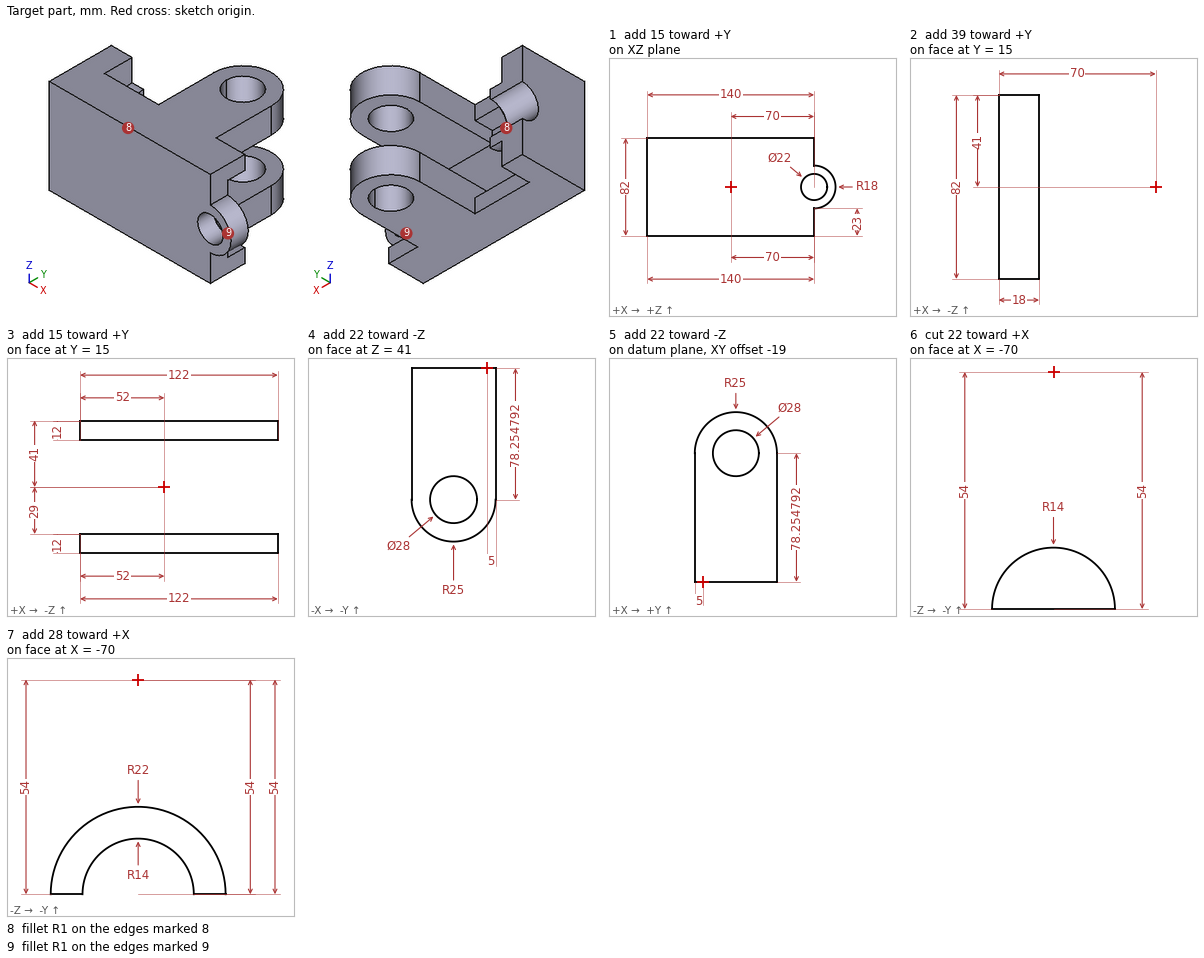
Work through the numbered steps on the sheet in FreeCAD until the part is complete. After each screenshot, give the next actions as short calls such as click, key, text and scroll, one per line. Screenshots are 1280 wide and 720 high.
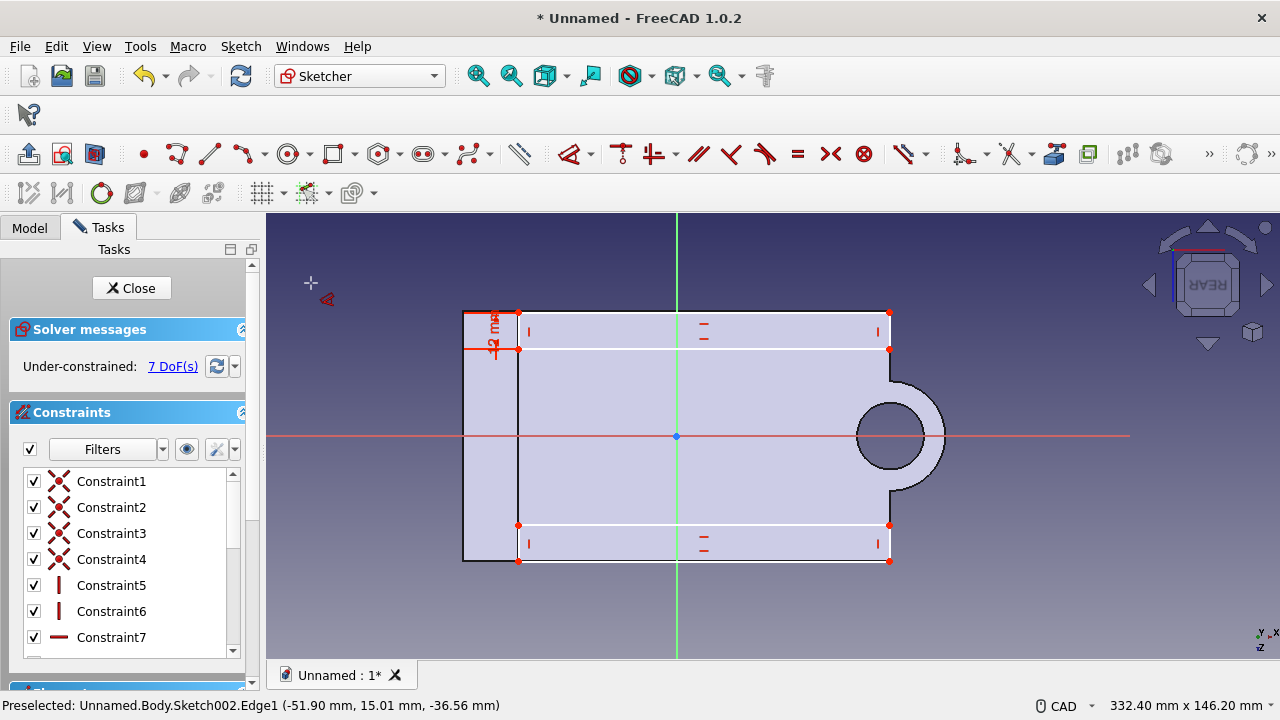
scroll(519, 536, up, 2)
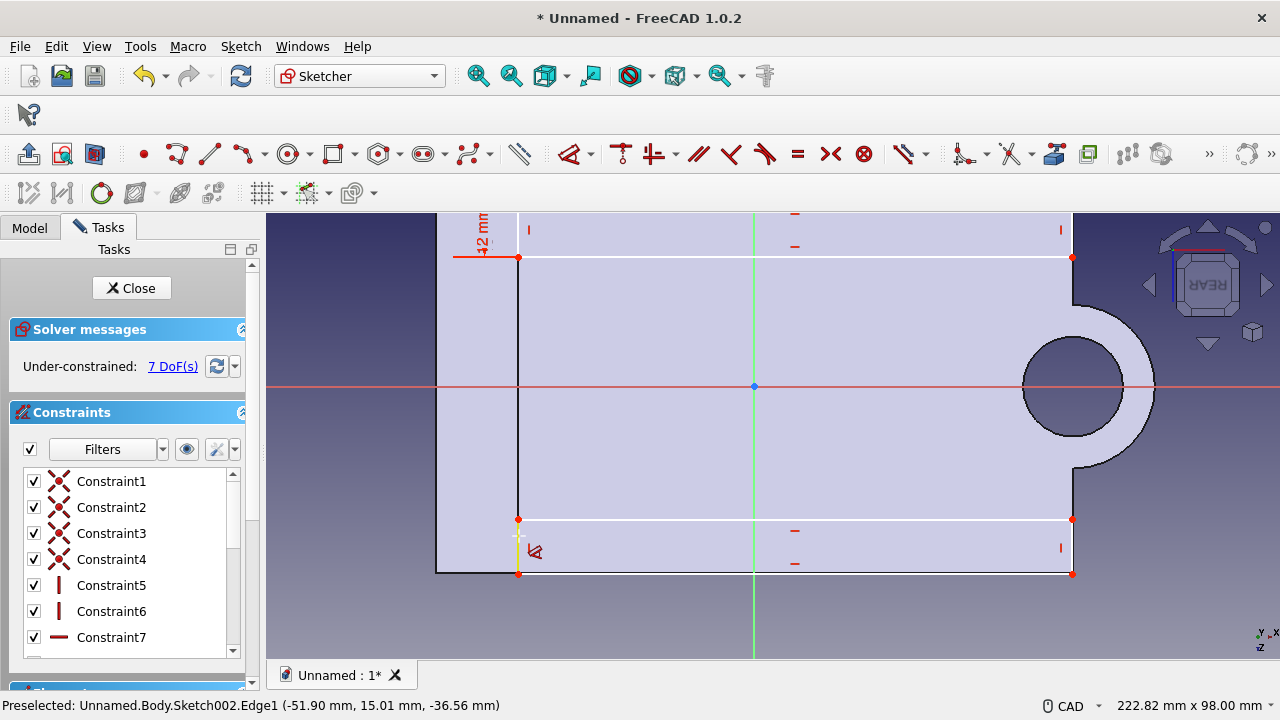
click(518, 536)
click(484, 547)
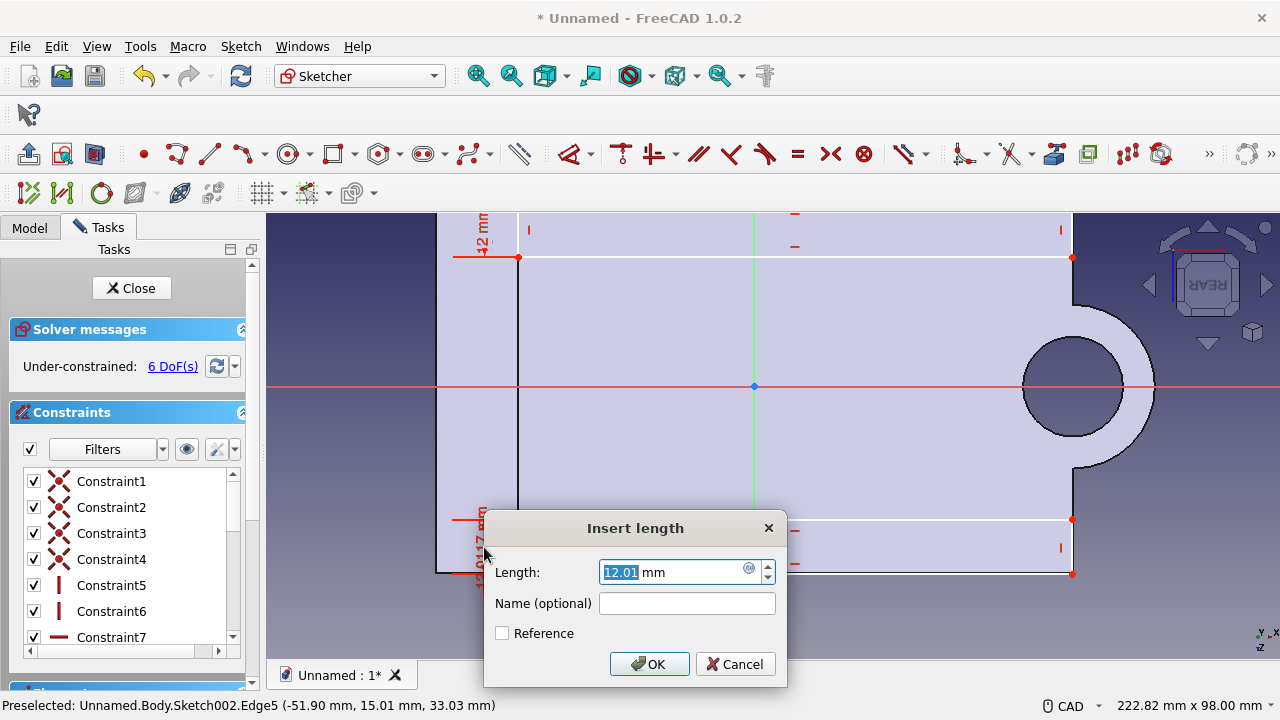
text(12)
key(Return)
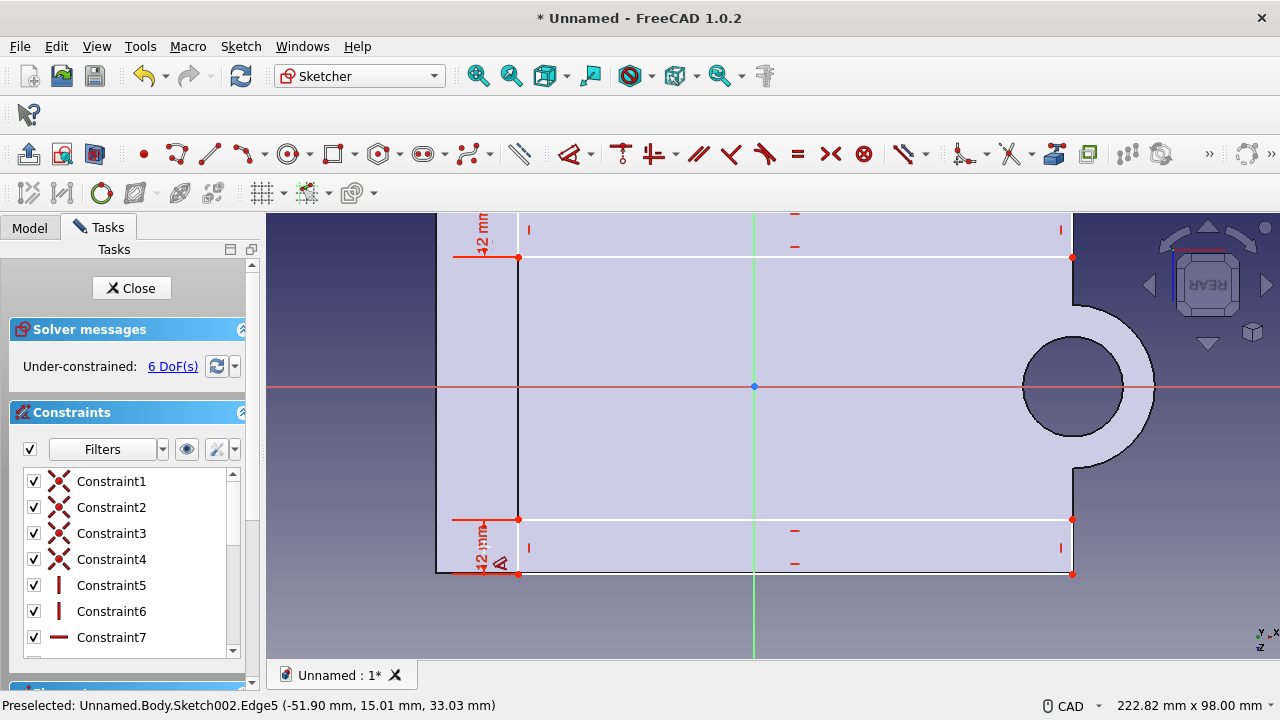
click(684, 257)
click(795, 291)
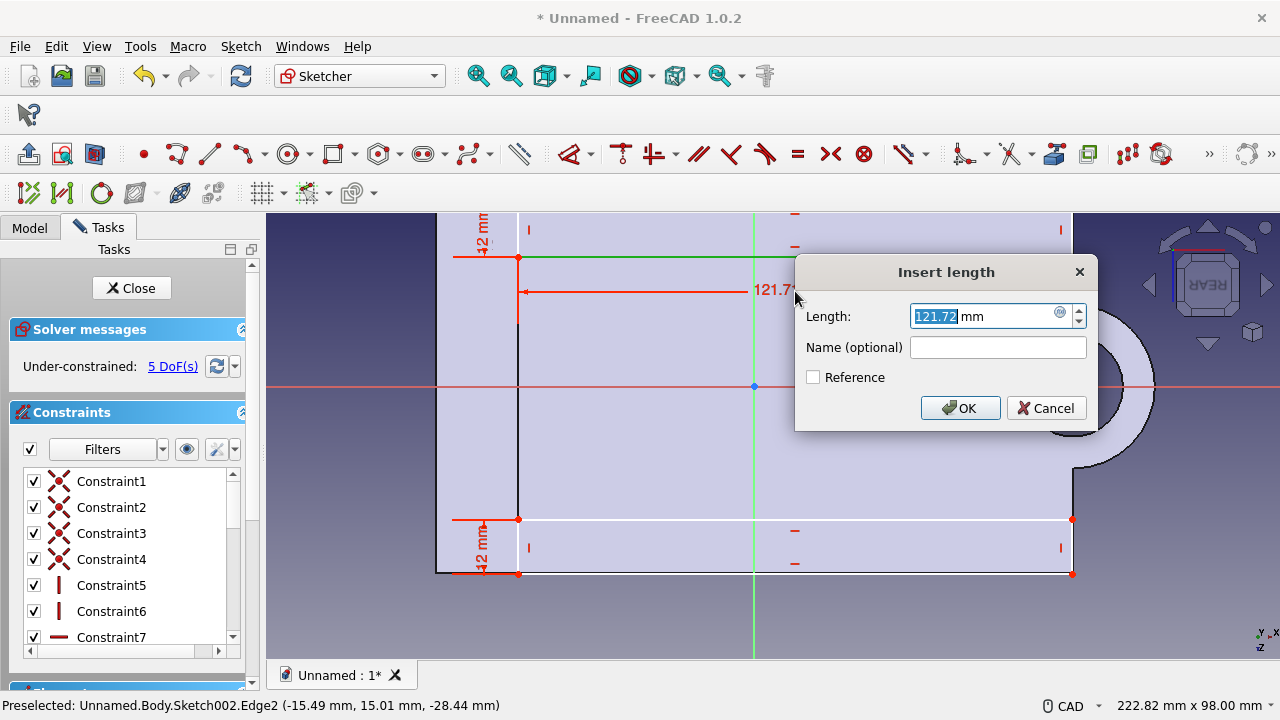
text(122)
key(Return)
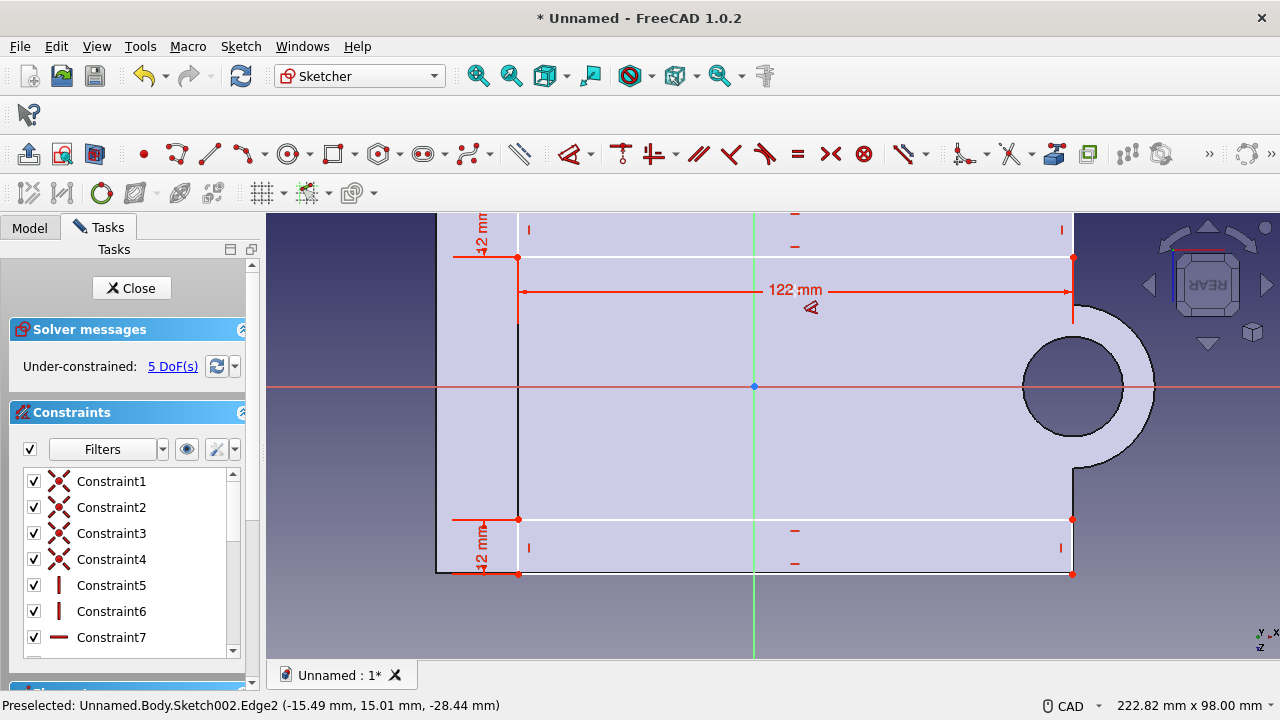
click(684, 574)
click(795, 608)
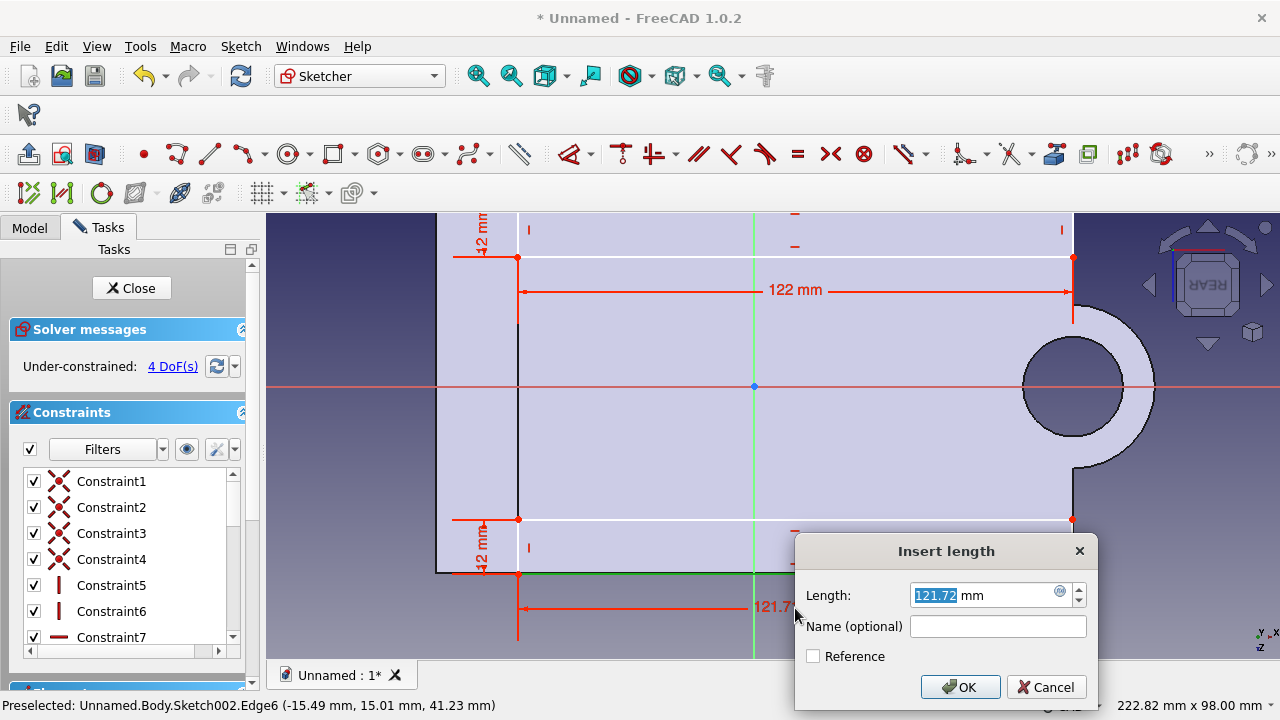
text(122)
key(Return)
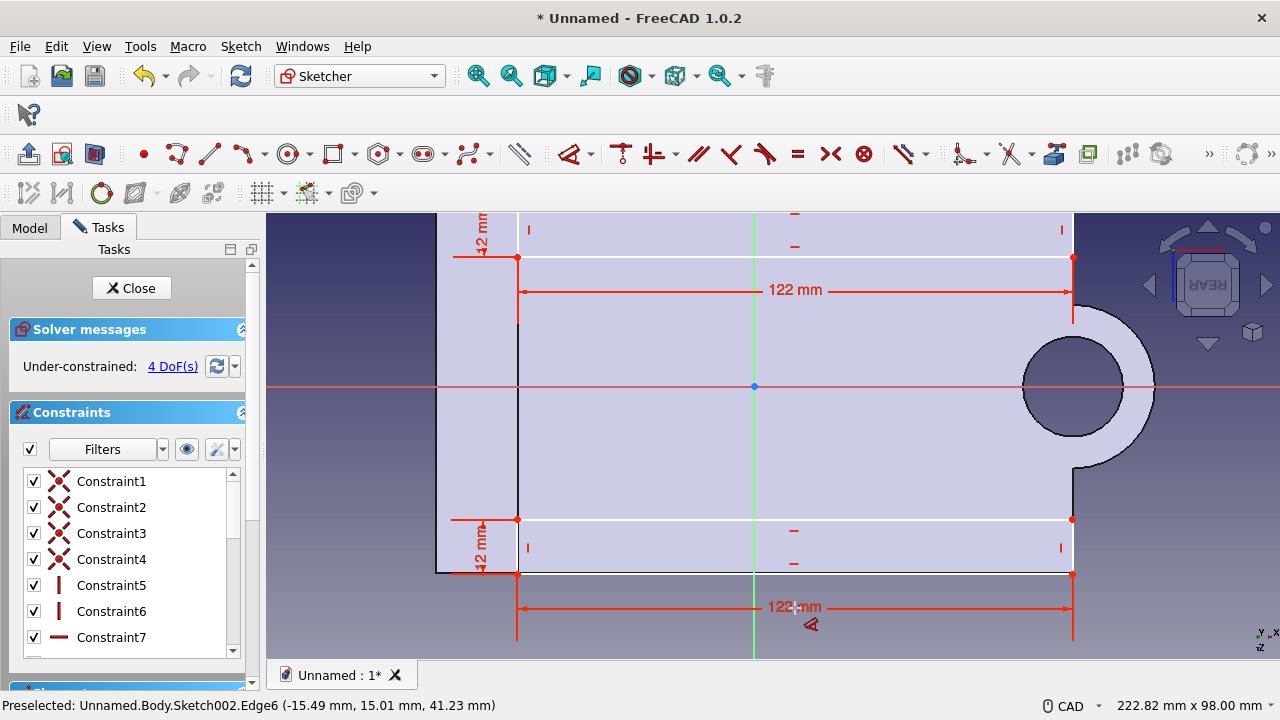
scroll(520, 536, down, 2)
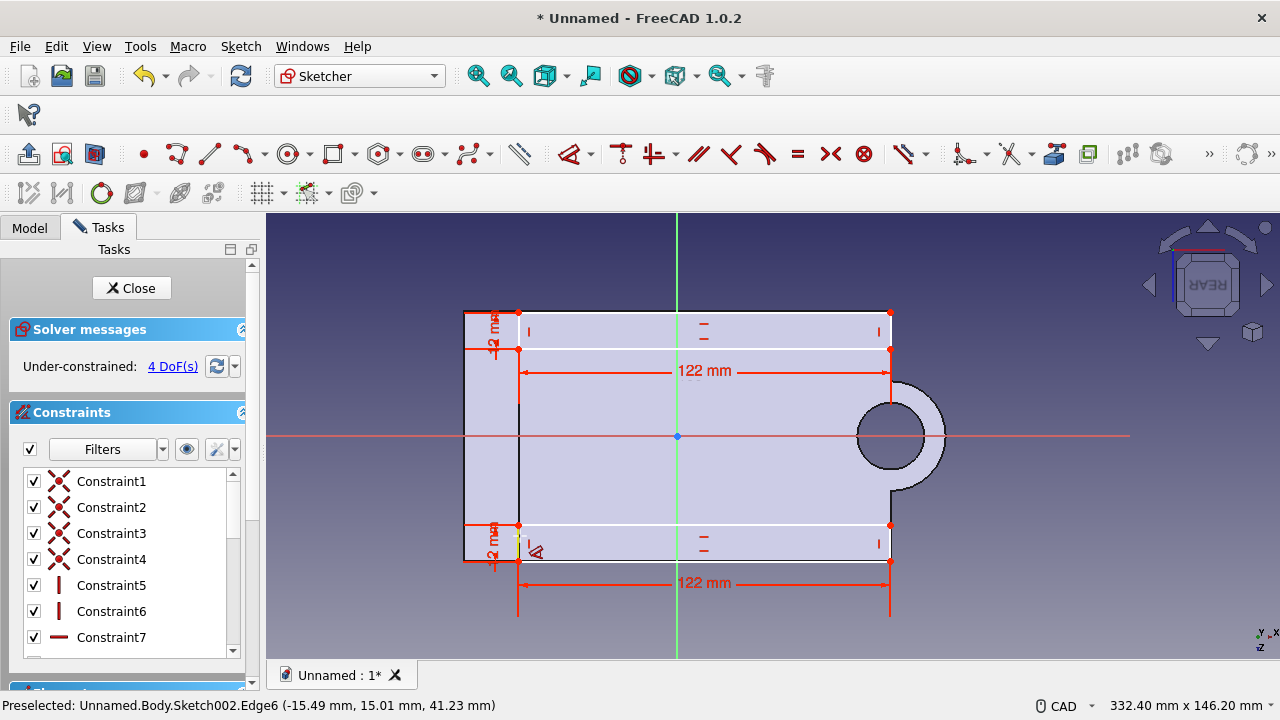
click(519, 313)
click(598, 279)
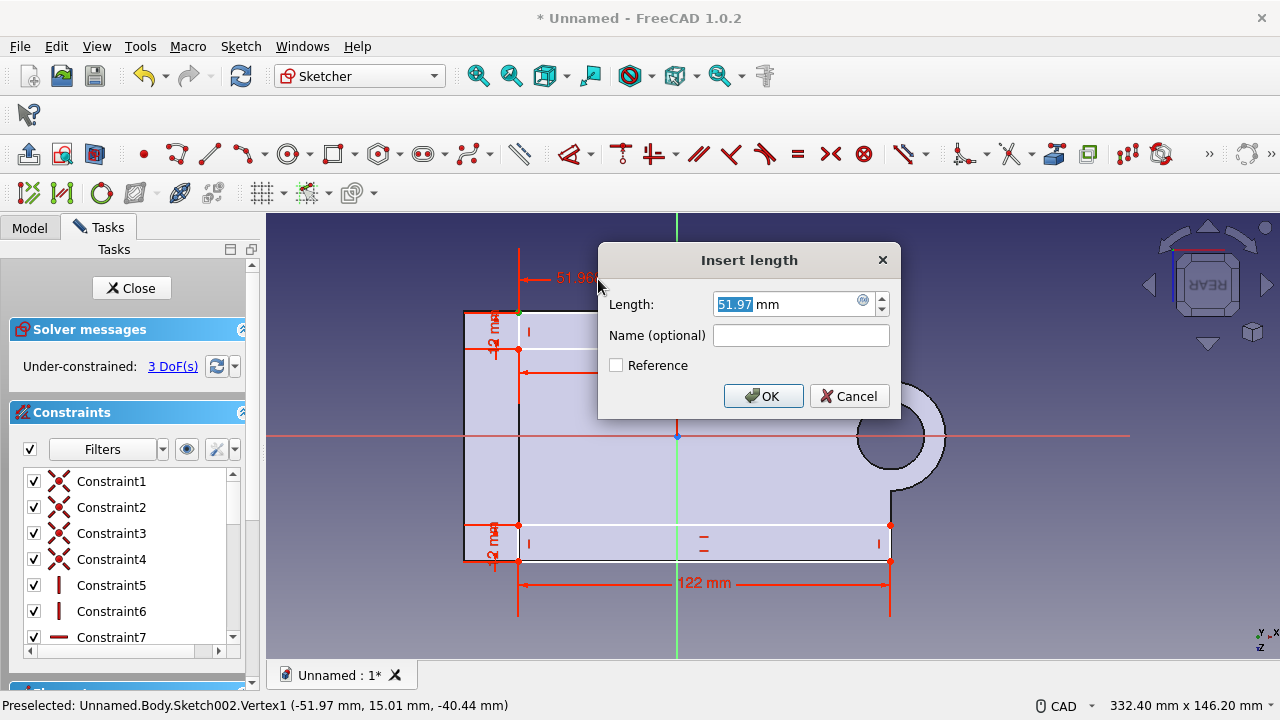
text(52)
key(Return)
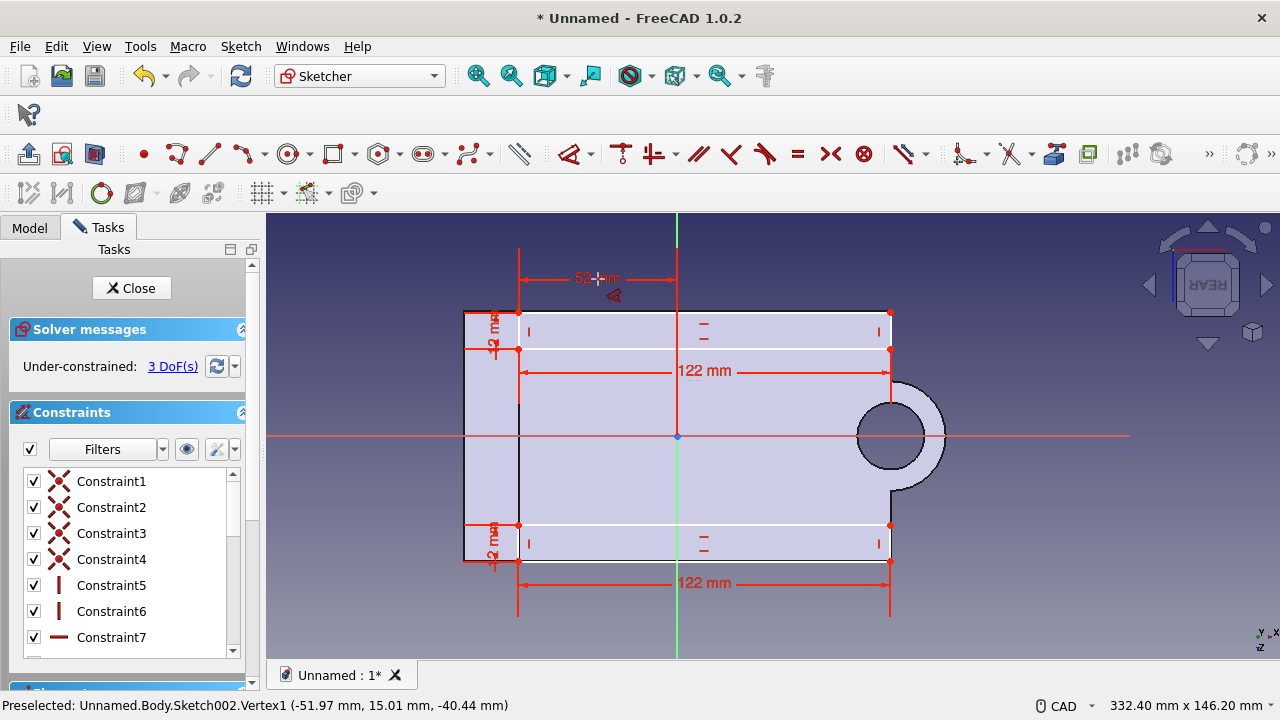
click(519, 313)
click(485, 374)